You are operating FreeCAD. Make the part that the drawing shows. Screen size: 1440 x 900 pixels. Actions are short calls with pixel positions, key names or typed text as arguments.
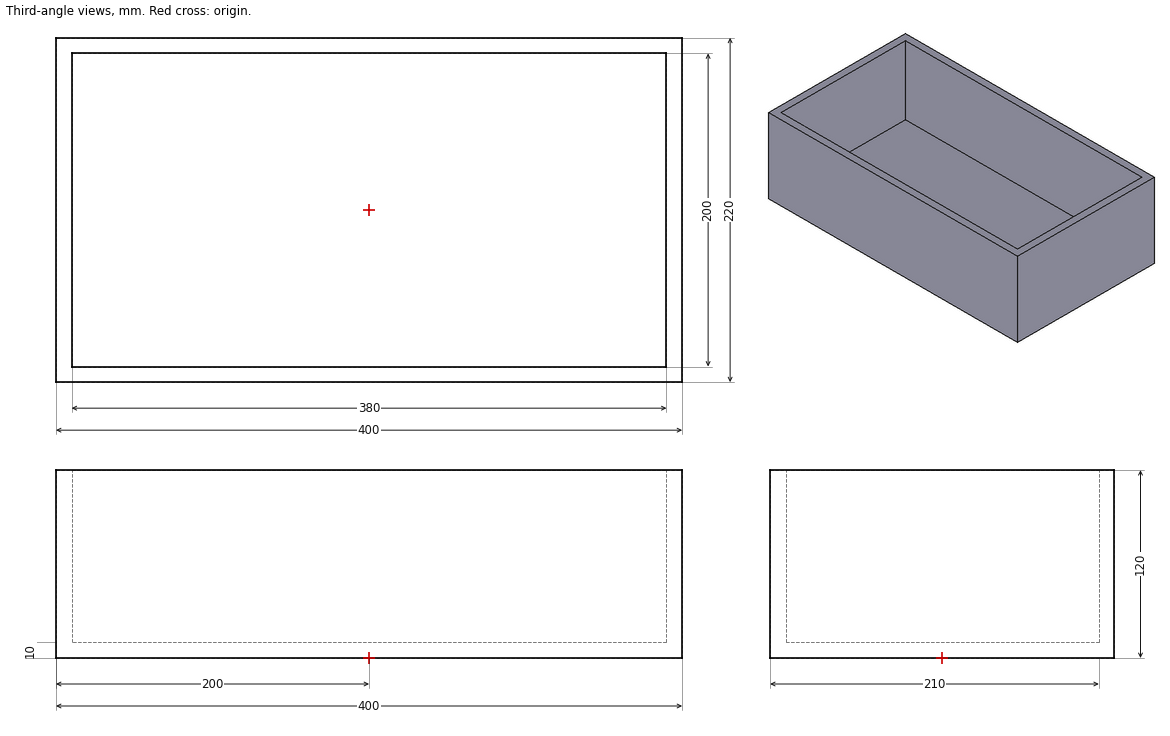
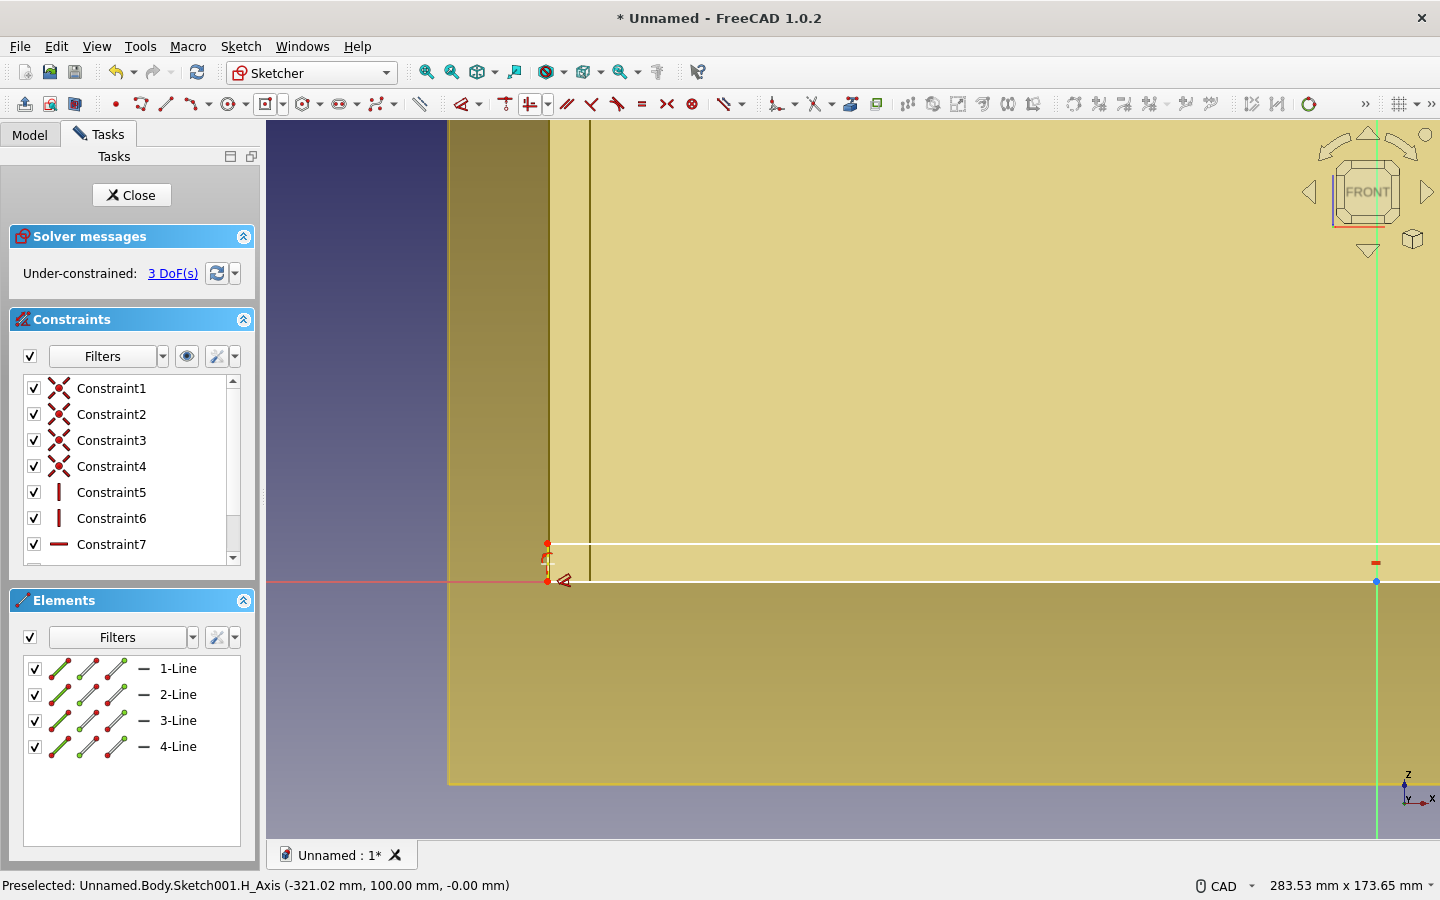
click(548, 563)
click(514, 563)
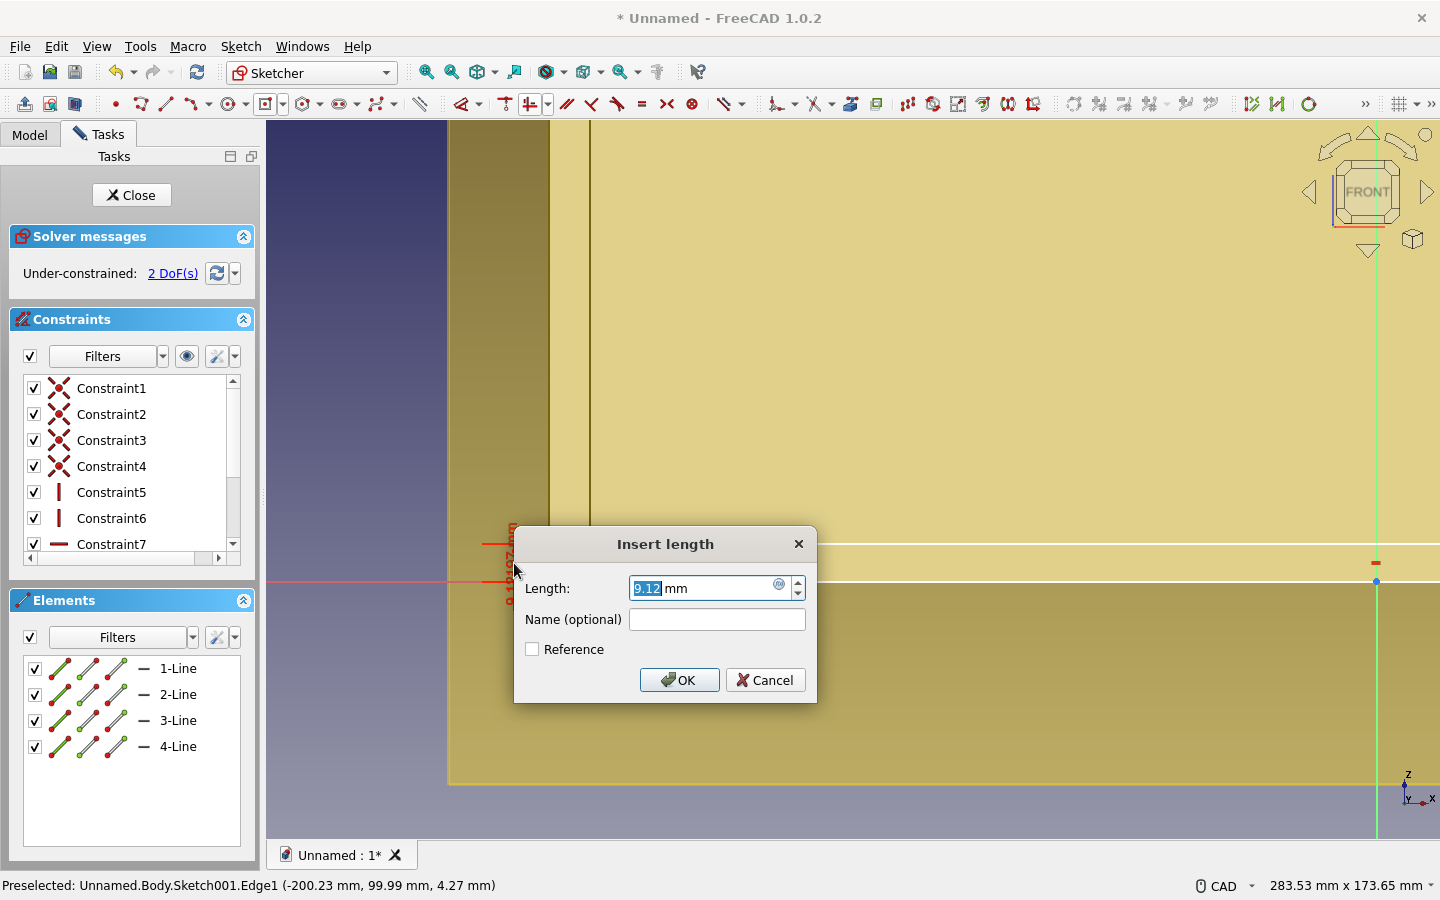
text(10)
key(Return)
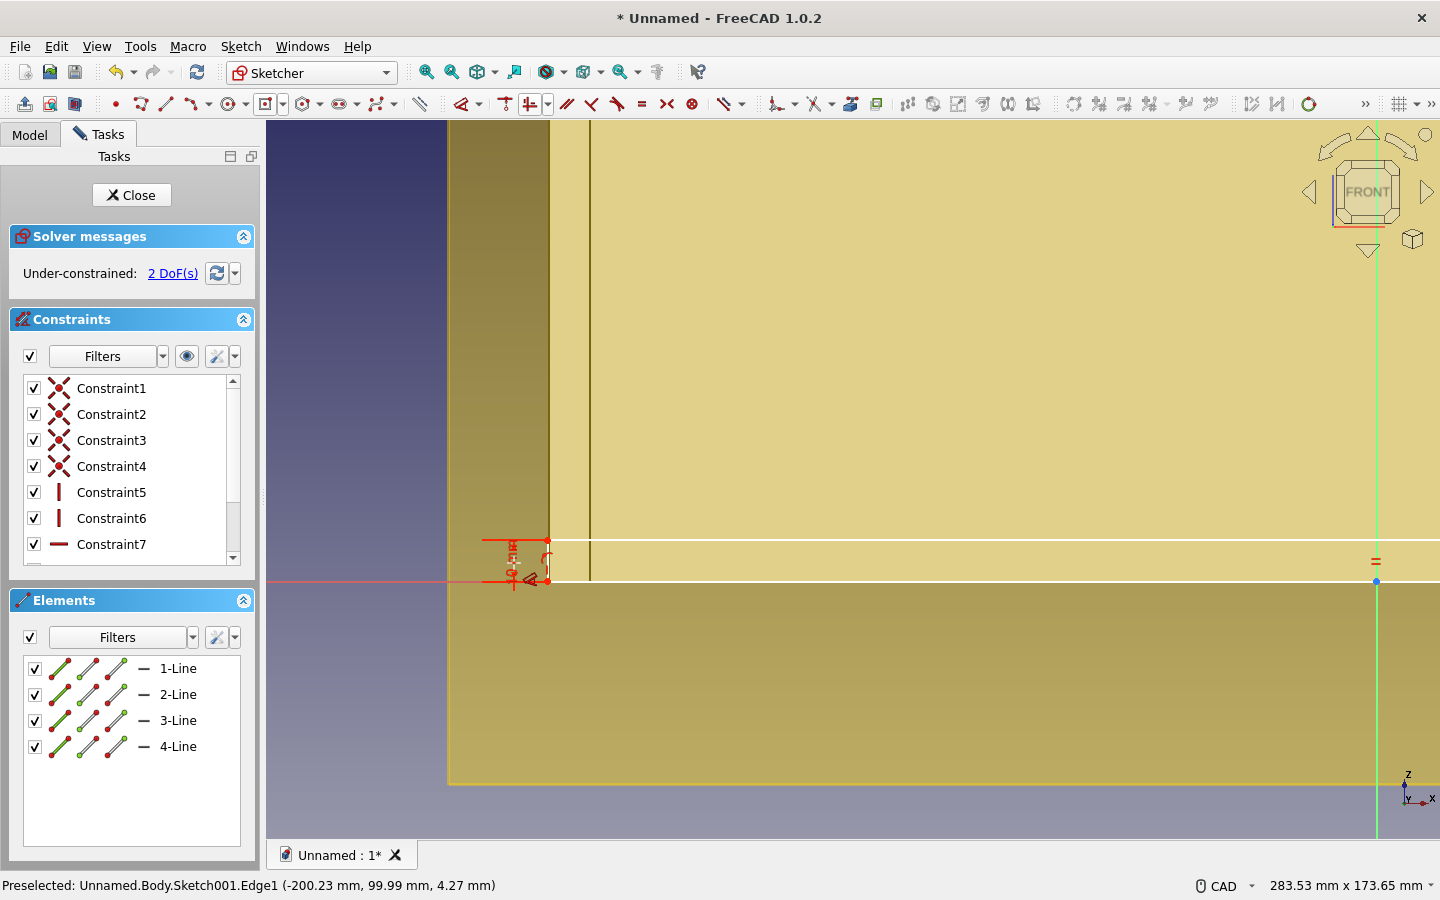
click(1045, 582)
click(911, 616)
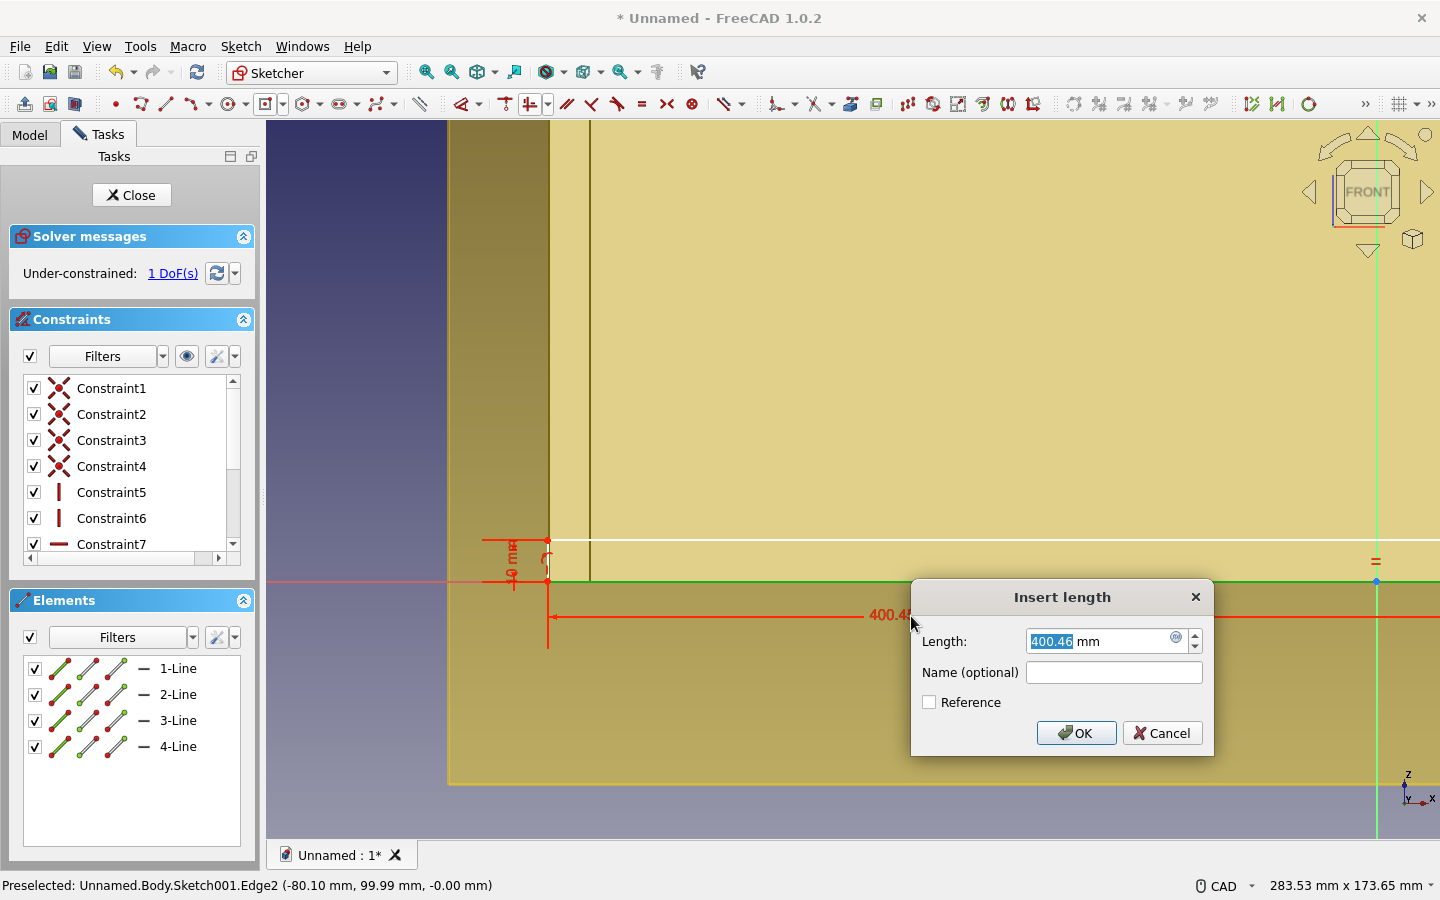
text(400)
key(Return)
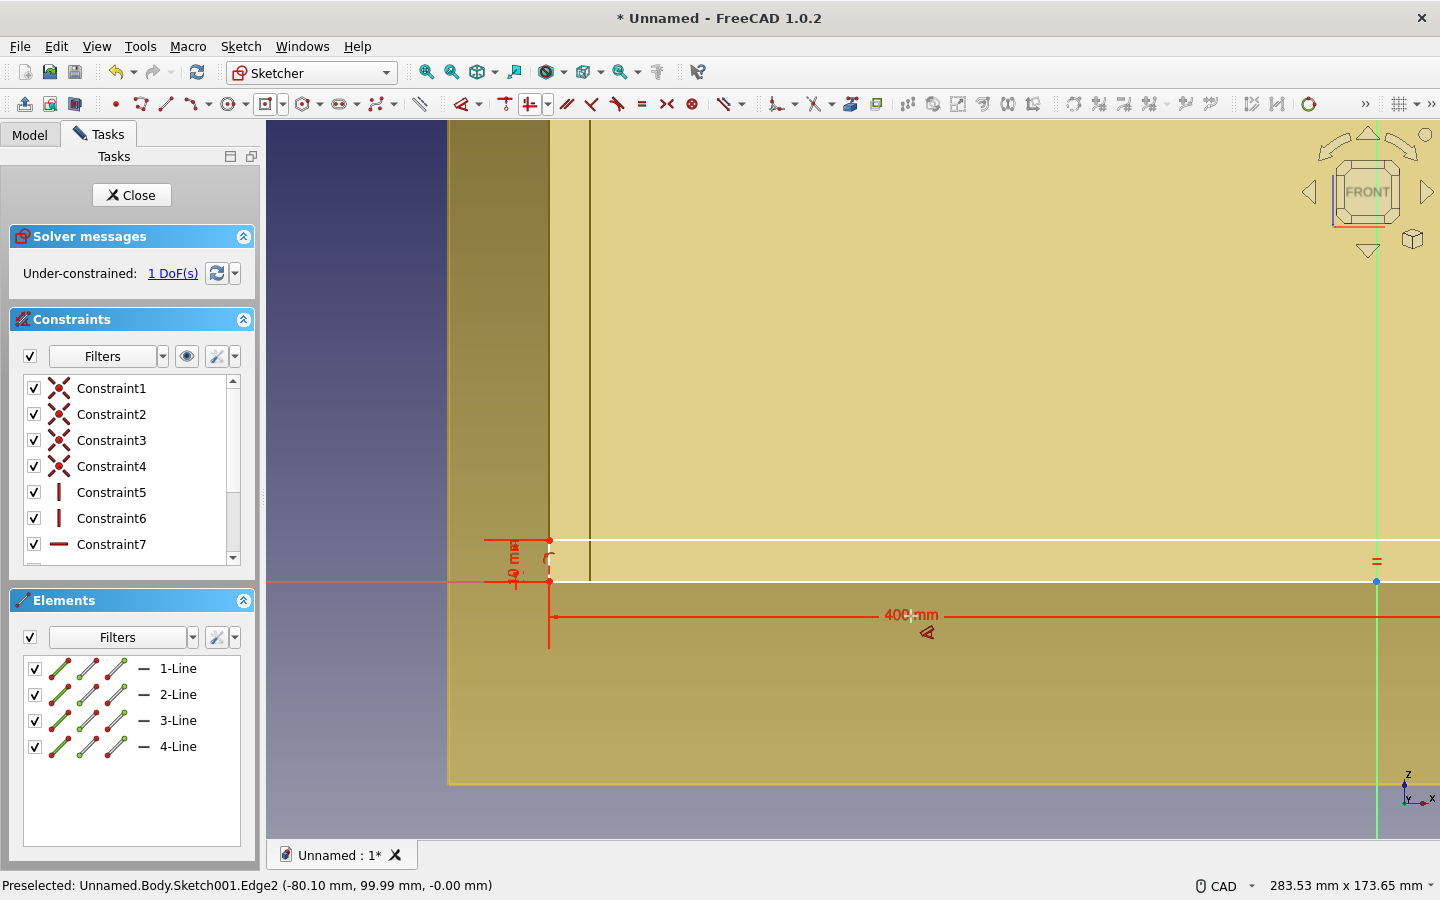
click(549, 540)
click(745, 616)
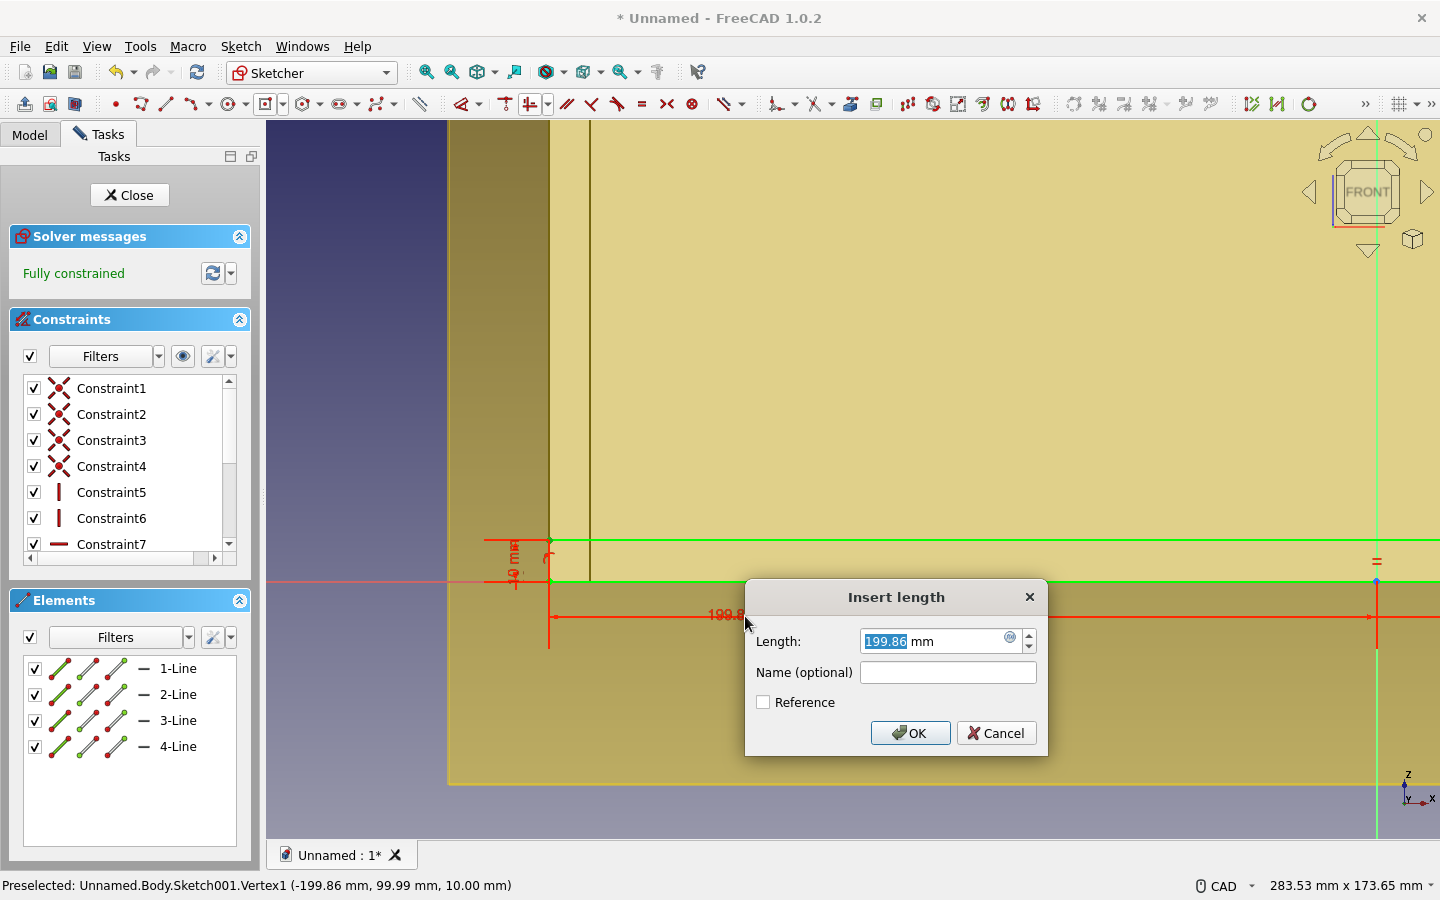
text(200)
key(Return)
key(Escape)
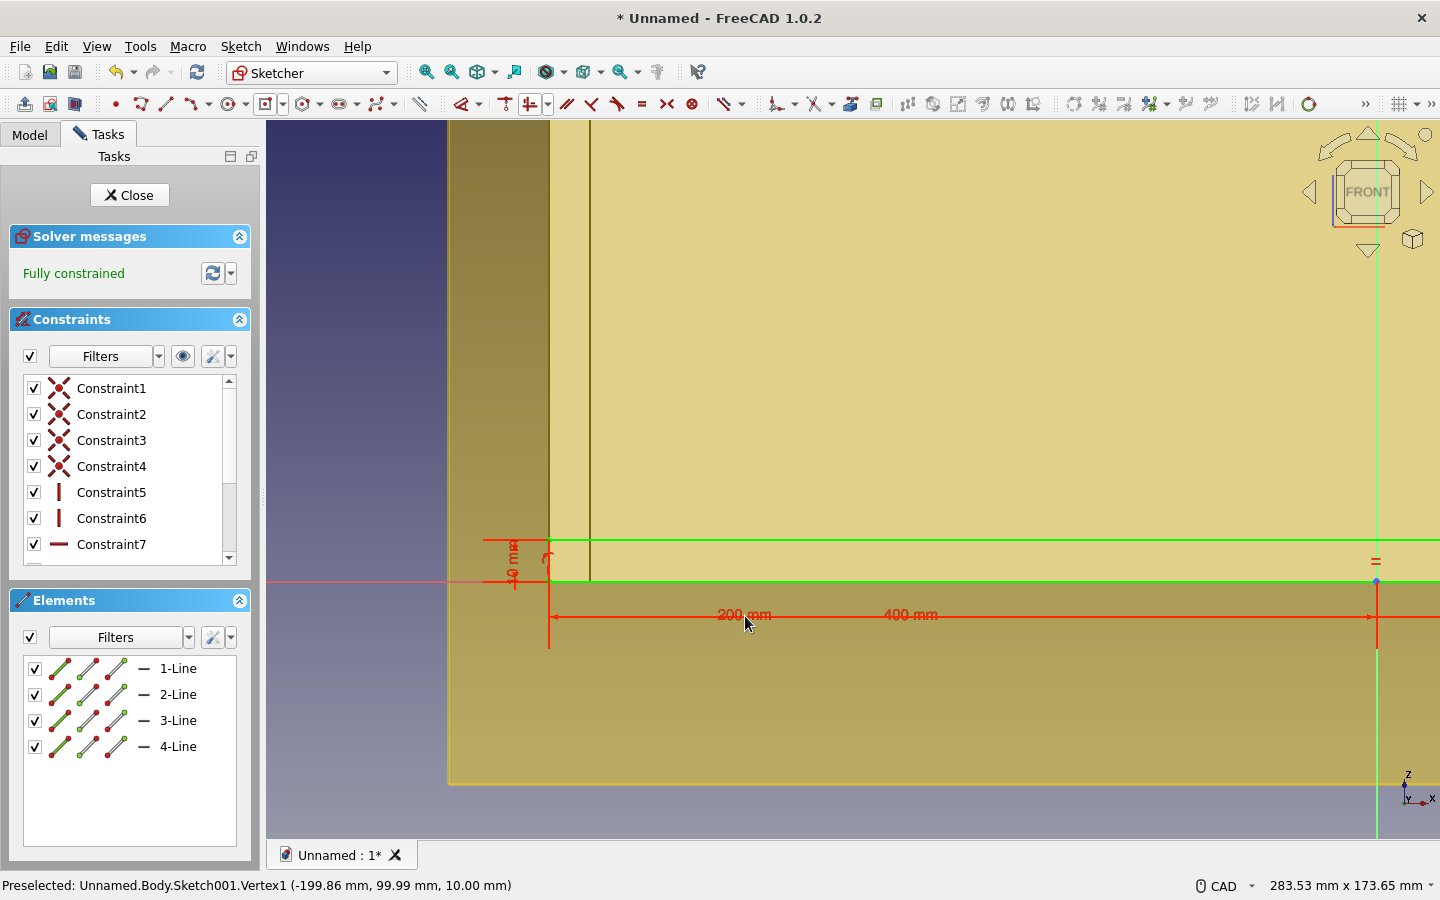
click(130, 195)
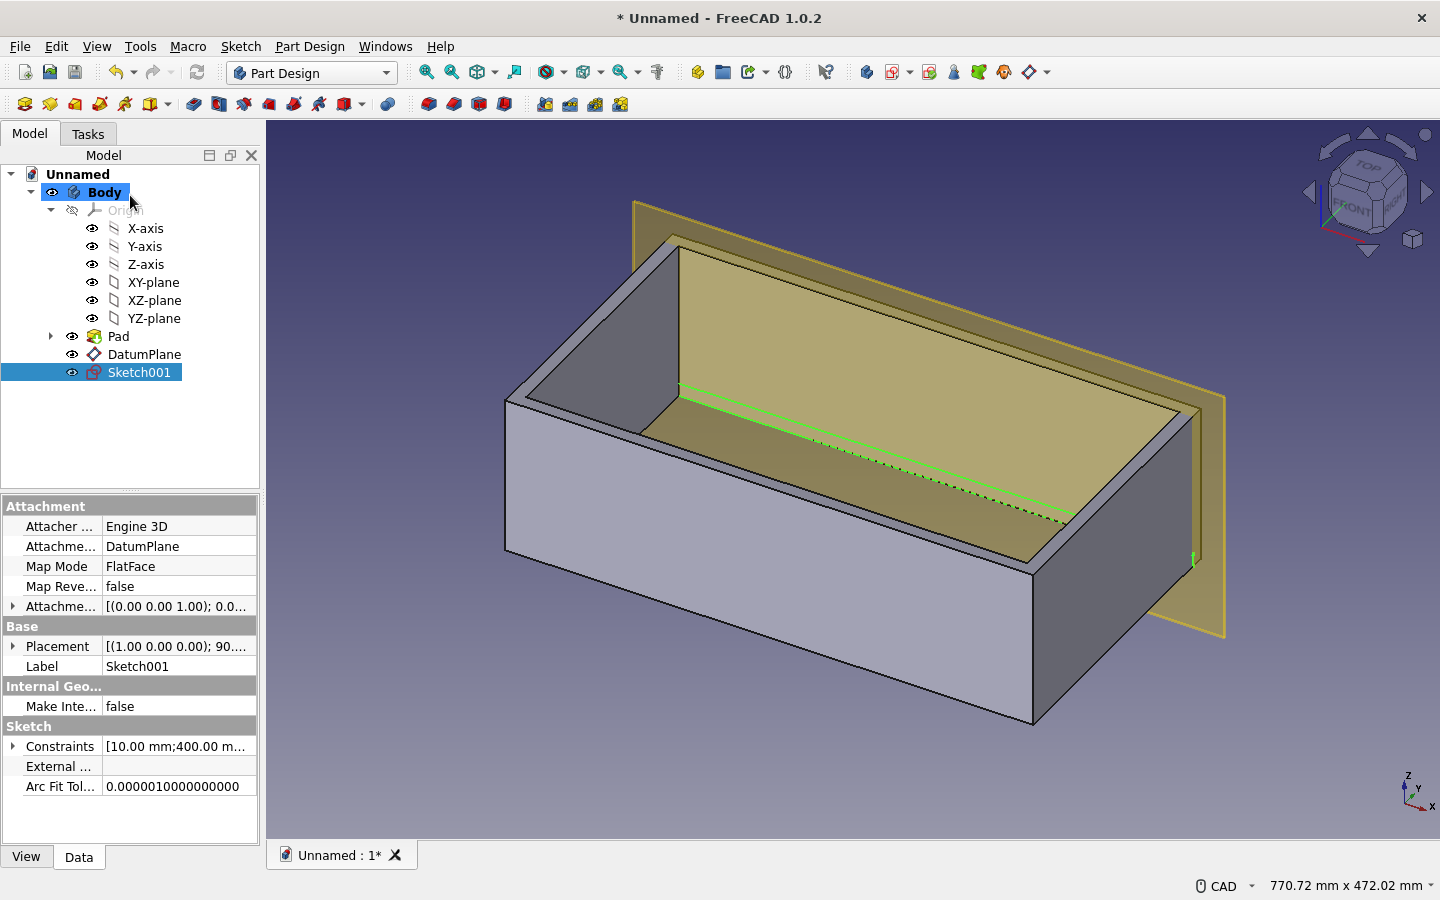
click(25, 104)